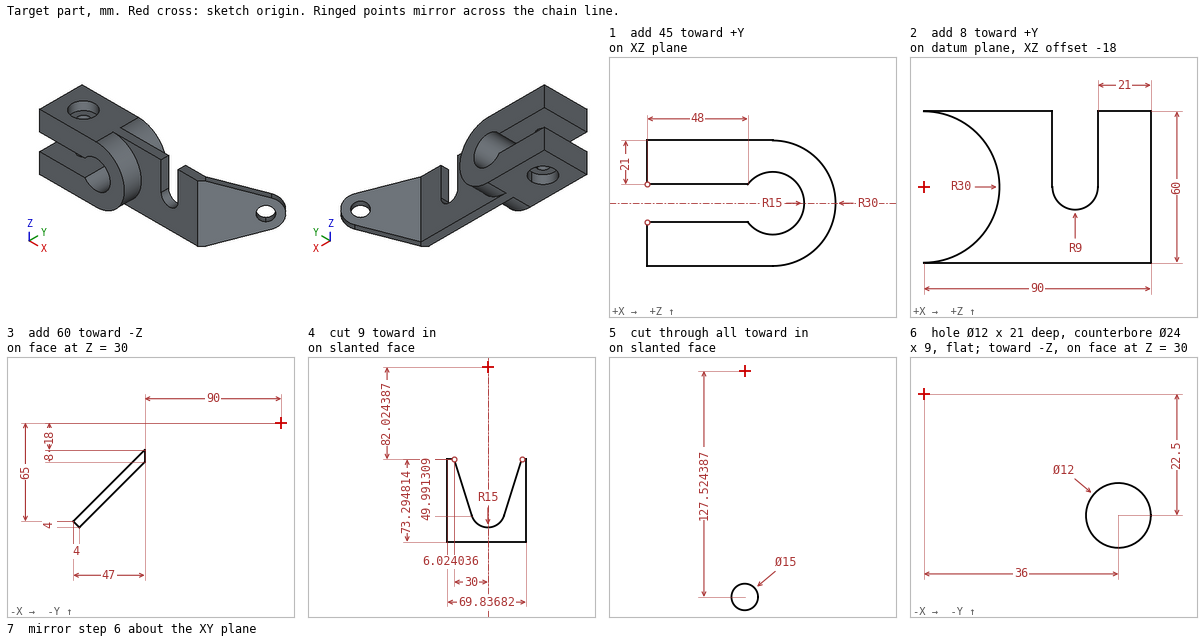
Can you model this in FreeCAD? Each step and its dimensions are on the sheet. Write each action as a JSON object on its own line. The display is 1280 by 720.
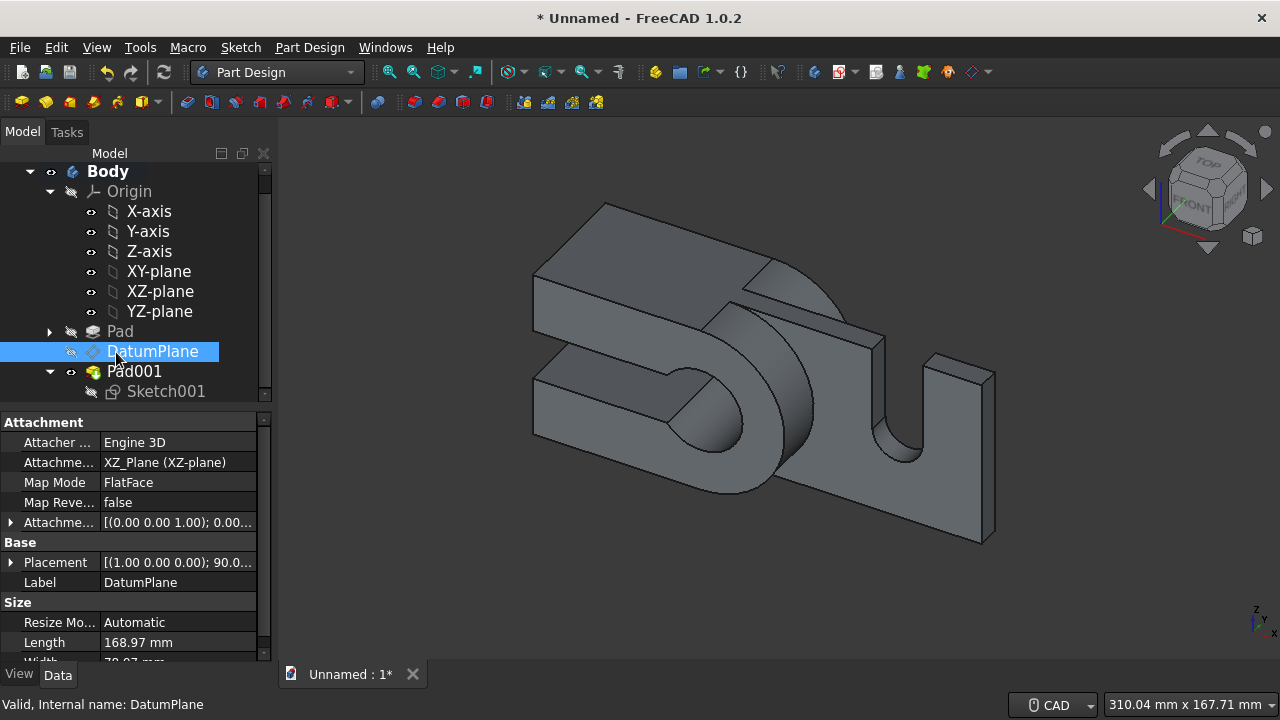
{"action": "left_click", "coordinate": [636, 260]}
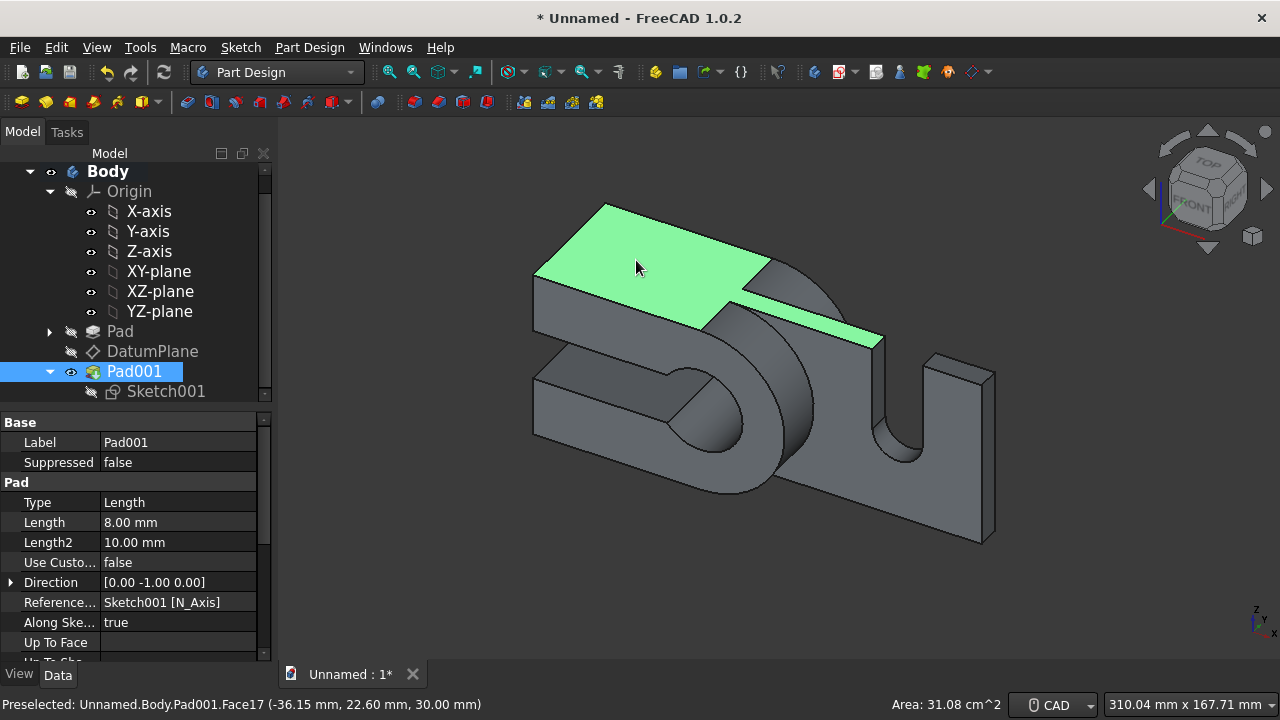
{"action": "left_click", "coordinate": [840, 72]}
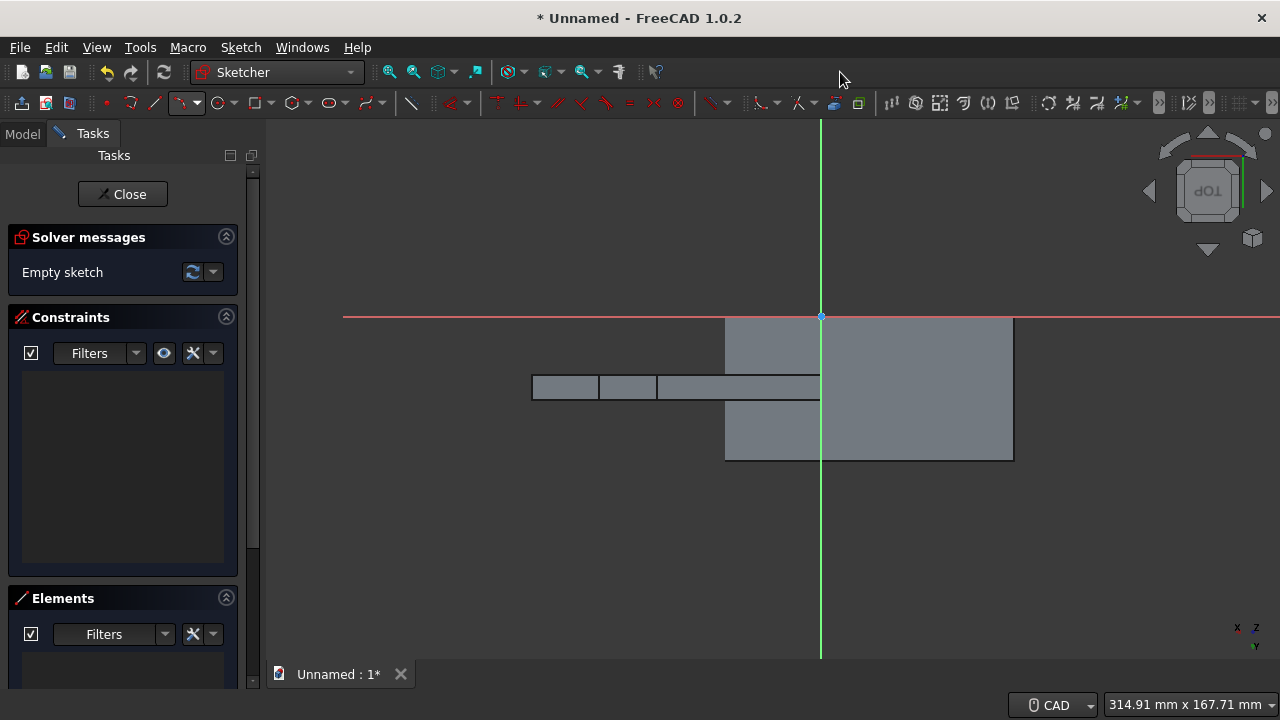
{"action": "scroll", "coordinate": [294, 512], "scroll_direction": "up", "scroll_amount": 4}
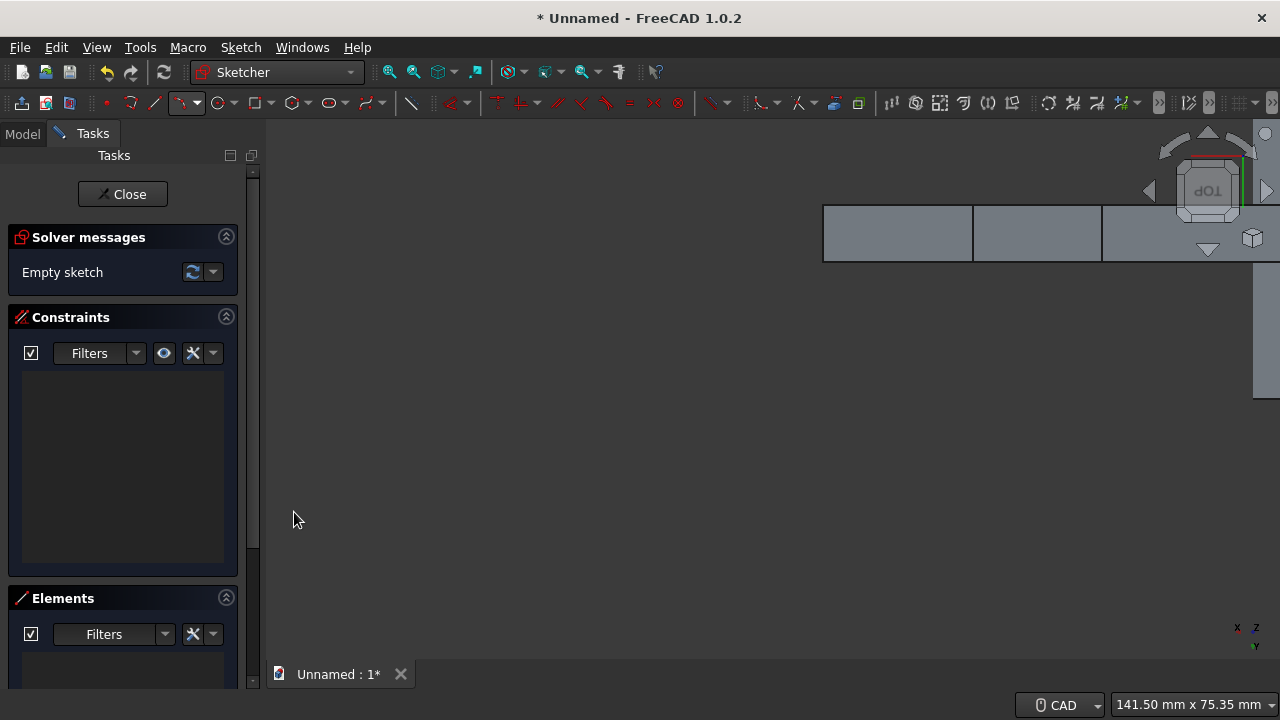
{"action": "left_click", "coordinate": [132, 104]}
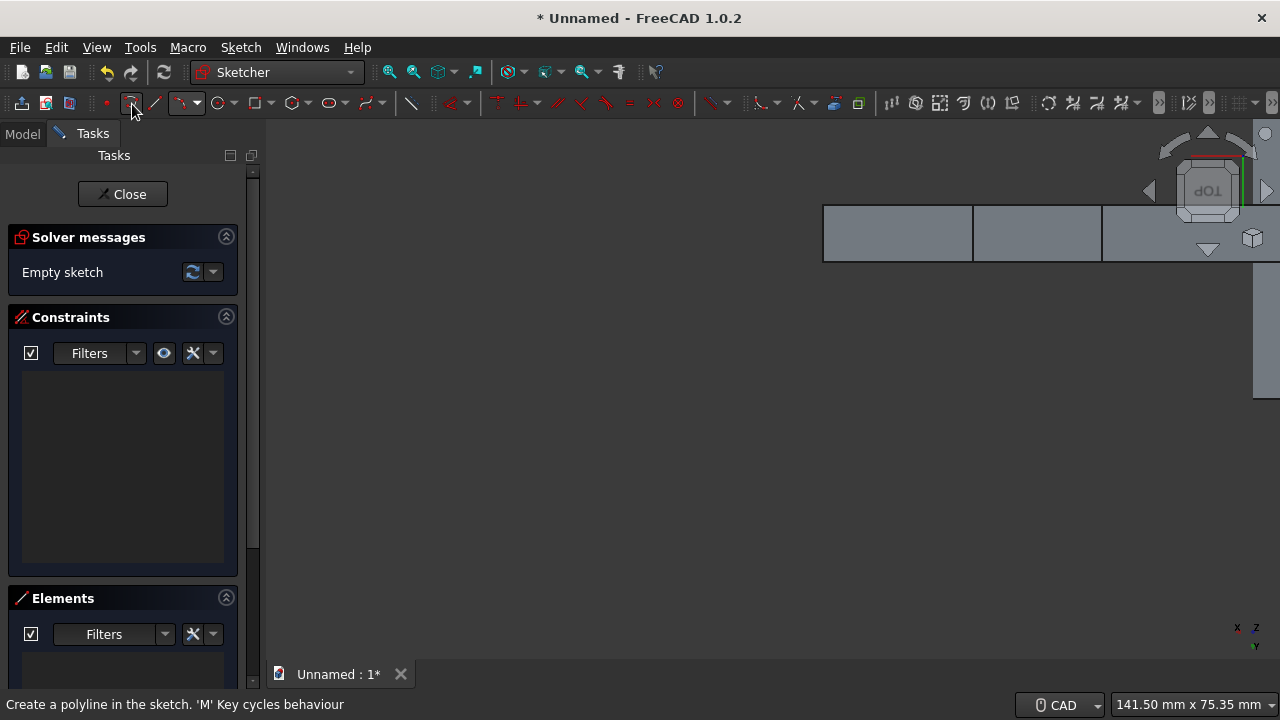
{"action": "left_click", "coordinate": [823, 205]}
{"action": "left_click", "coordinate": [486, 542]}
{"action": "left_click", "coordinate": [514, 571]}
{"action": "left_click", "coordinate": [823, 262]}
{"action": "left_click", "coordinate": [823, 206]}
{"action": "key", "text": "Escape"}
{"action": "key", "text": "Escape"}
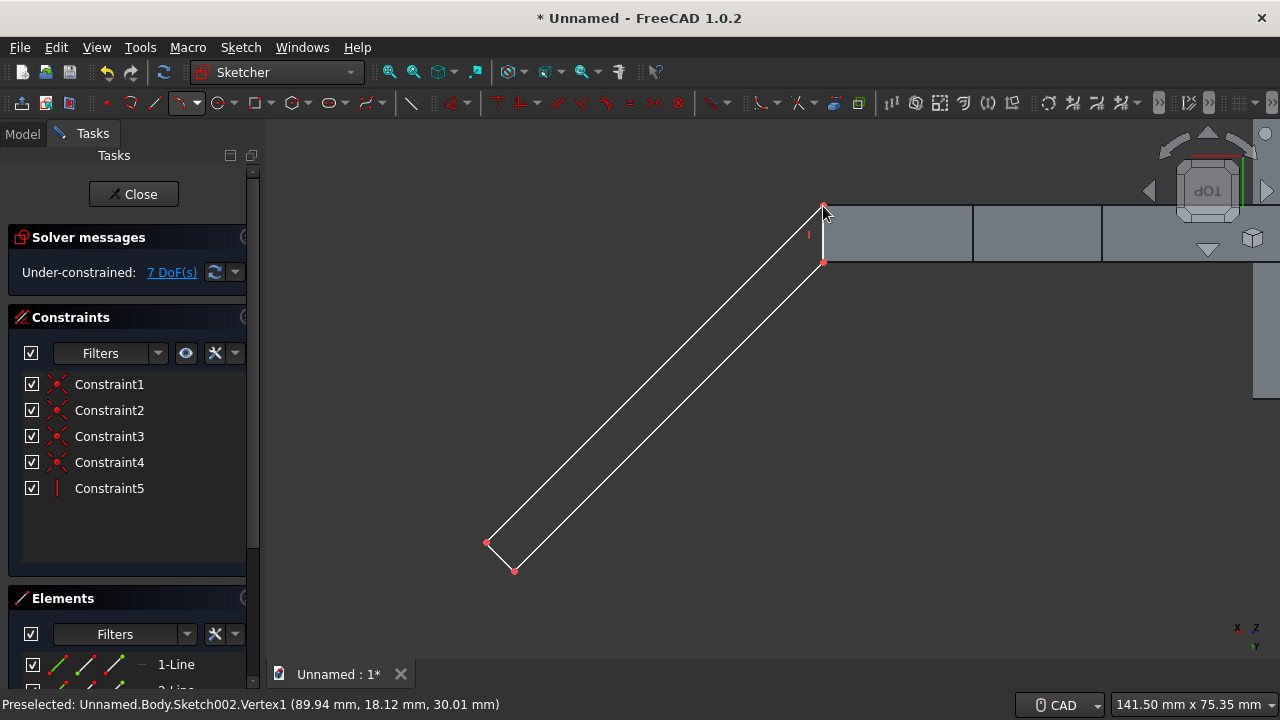
{"action": "left_click", "coordinate": [450, 104]}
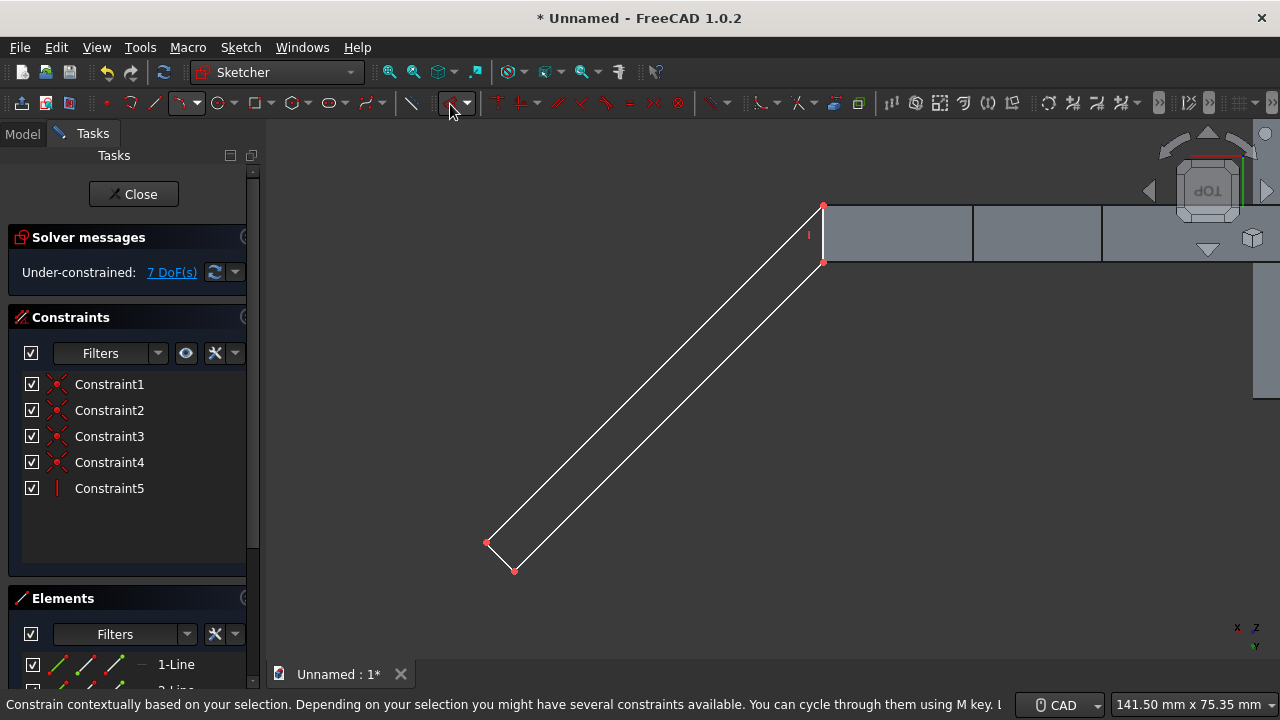
{"action": "left_click", "coordinate": [823, 246]}
{"action": "left_click", "coordinate": [857, 234]}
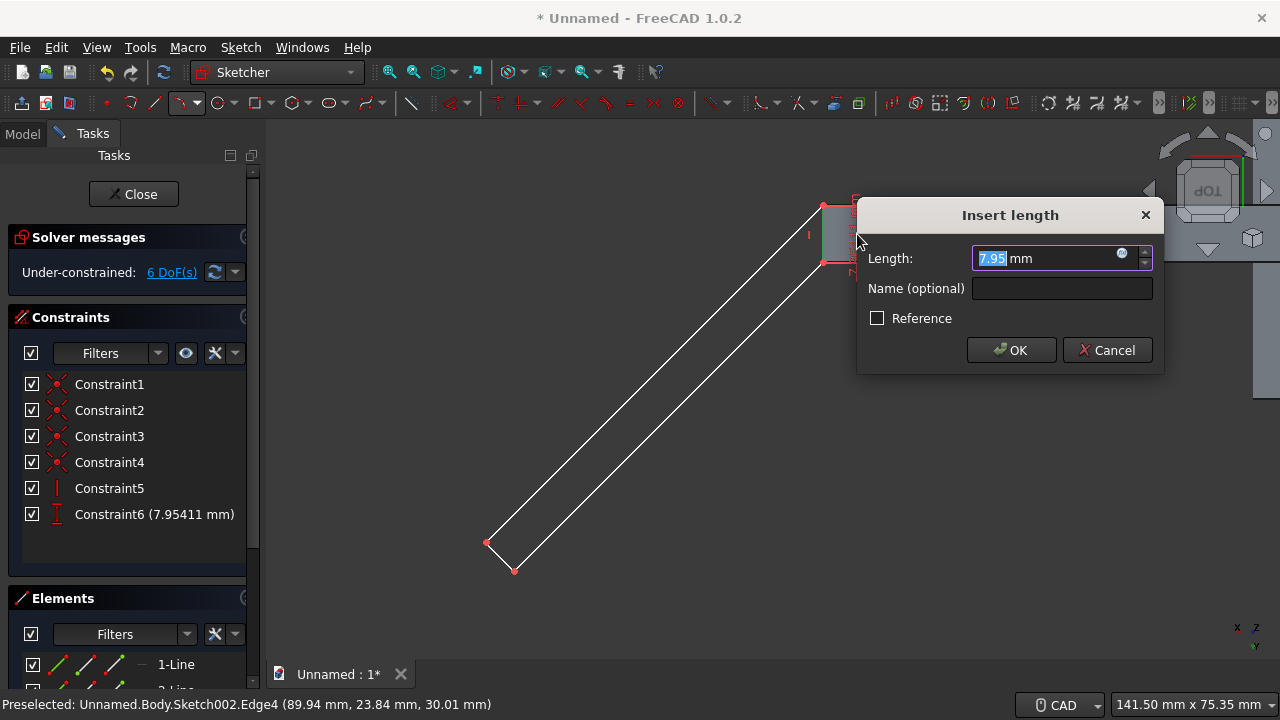
{"action": "type", "text": "8"}
{"action": "key", "text": "Return"}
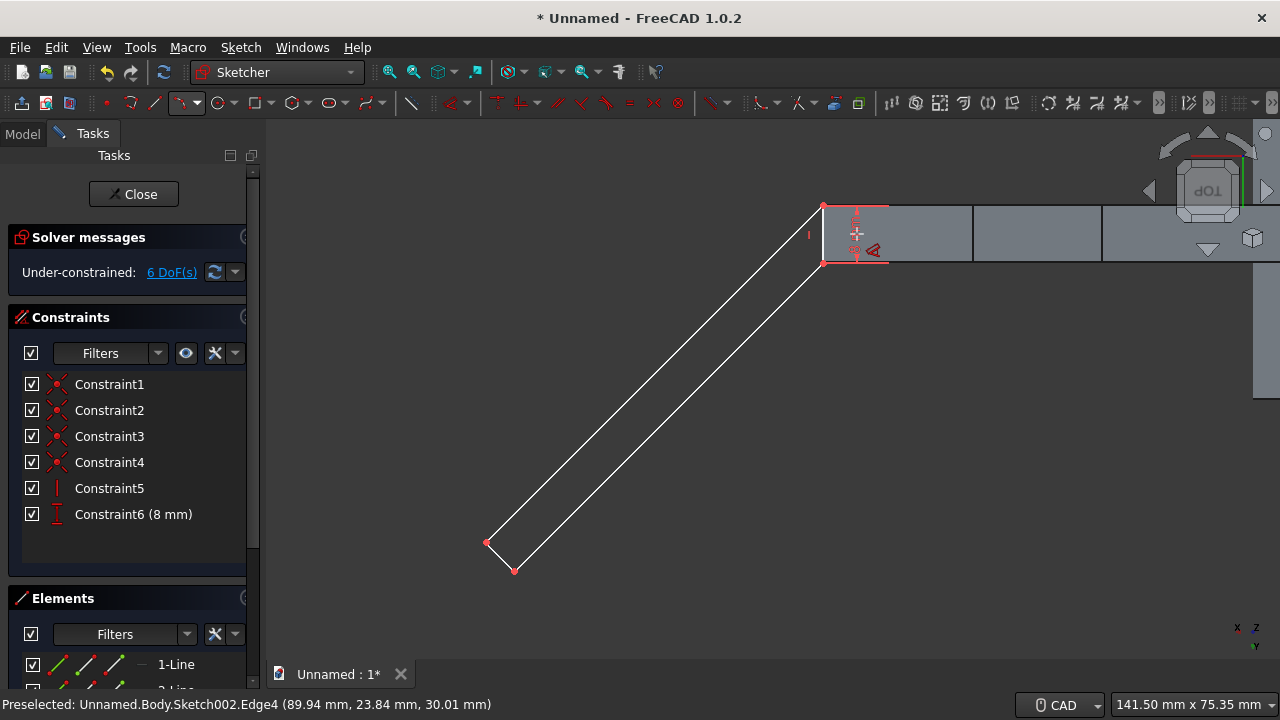
{"action": "scroll", "coordinate": [494, 552], "scroll_direction": "up", "scroll_amount": 2}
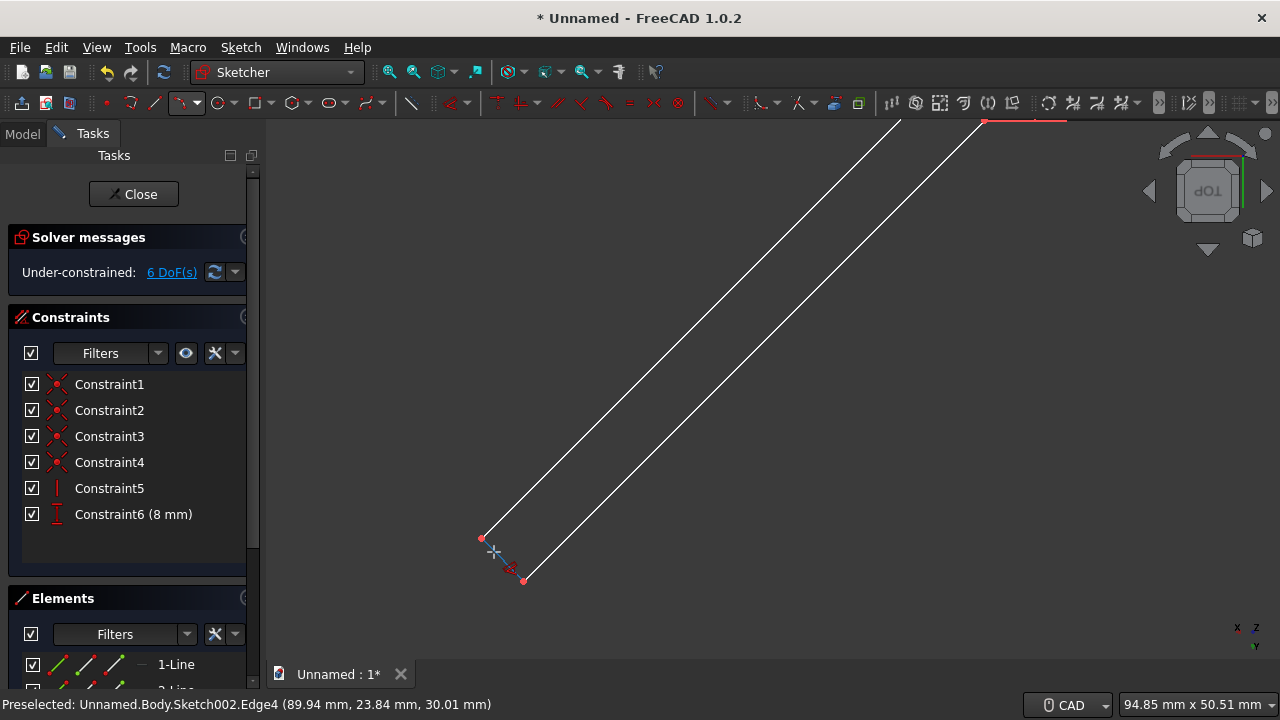
{"action": "left_click", "coordinate": [494, 551]}
{"action": "left_click", "coordinate": [503, 615]}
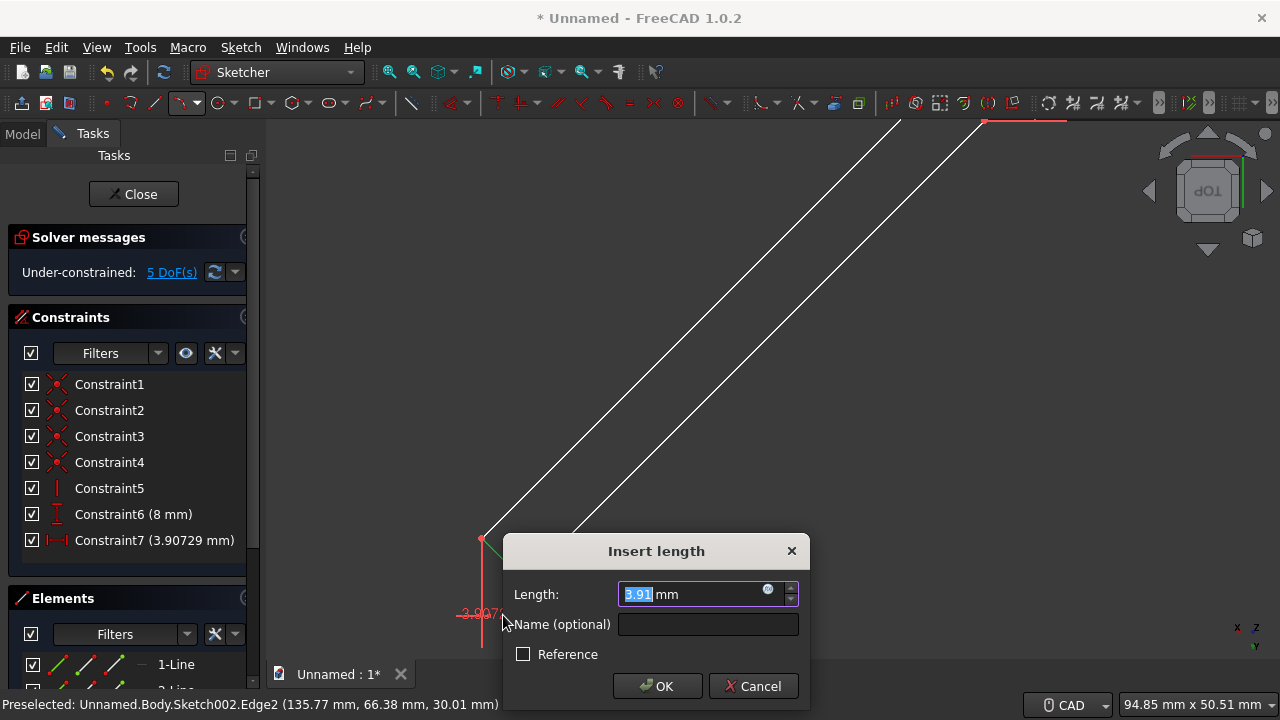
{"action": "type", "text": "4"}
{"action": "key", "text": "Return"}